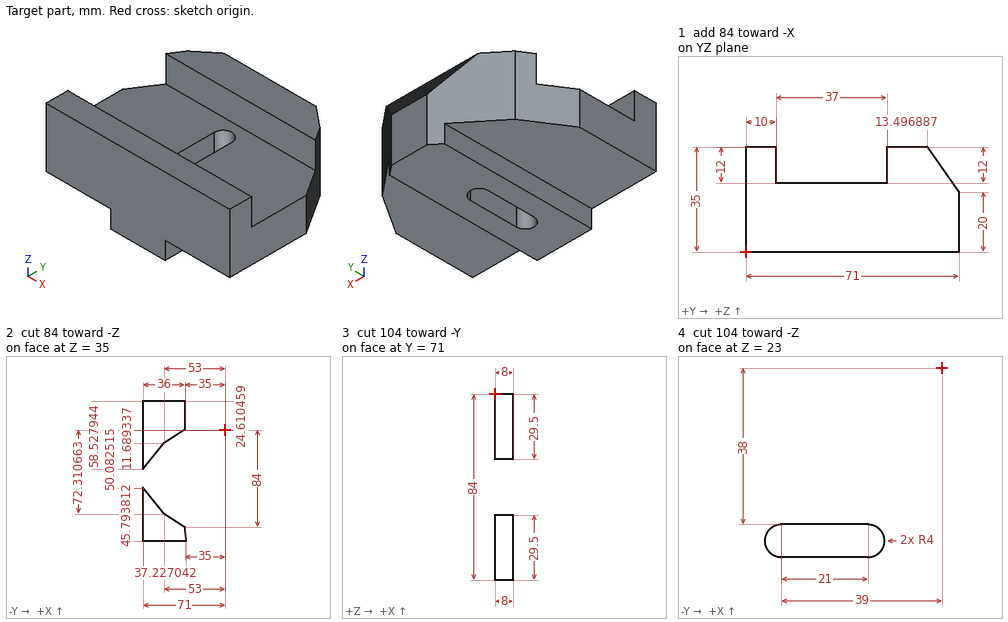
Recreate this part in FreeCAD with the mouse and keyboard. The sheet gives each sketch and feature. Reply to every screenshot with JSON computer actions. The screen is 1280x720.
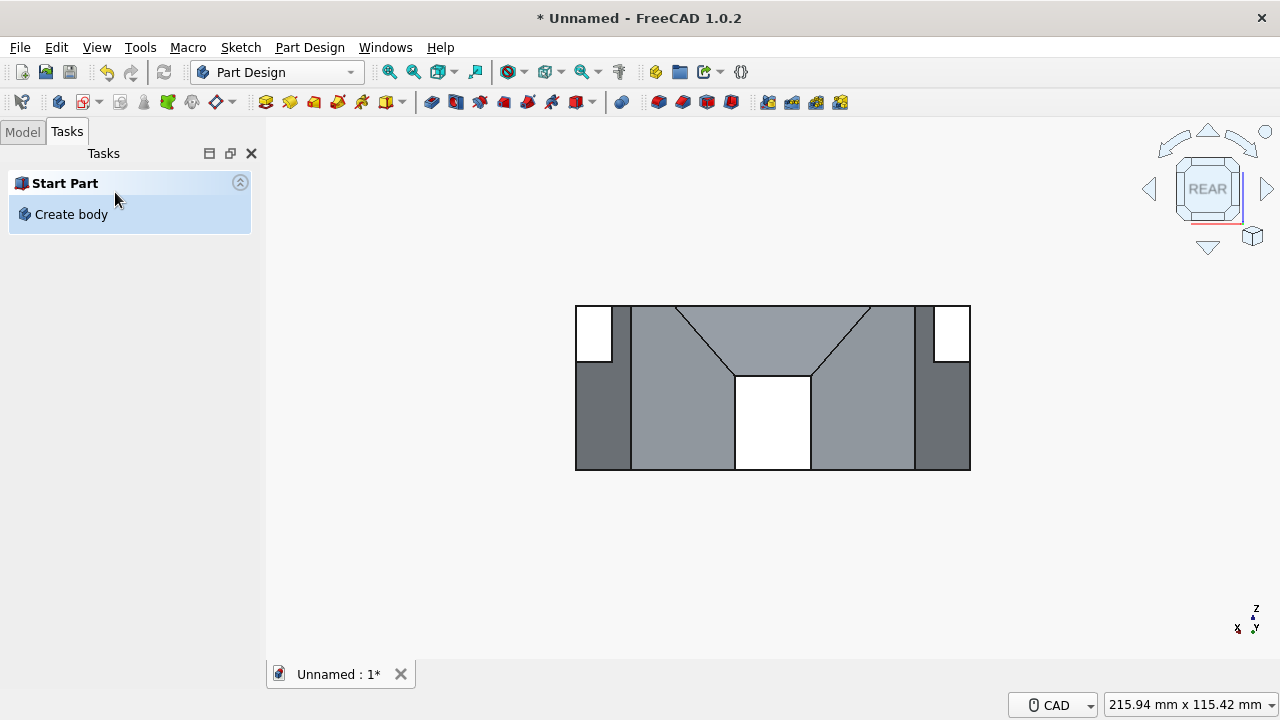
{"action": "left_click", "coordinate": [390, 72]}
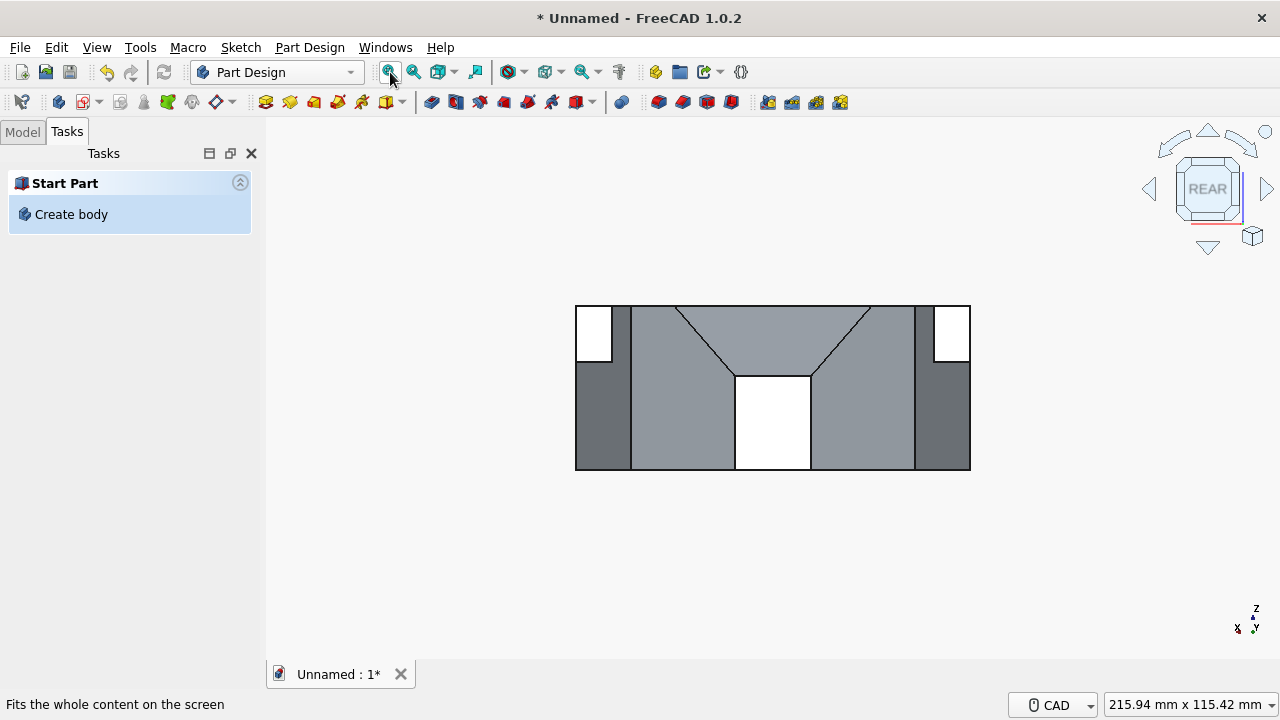
{"action": "left_click", "coordinate": [773, 422]}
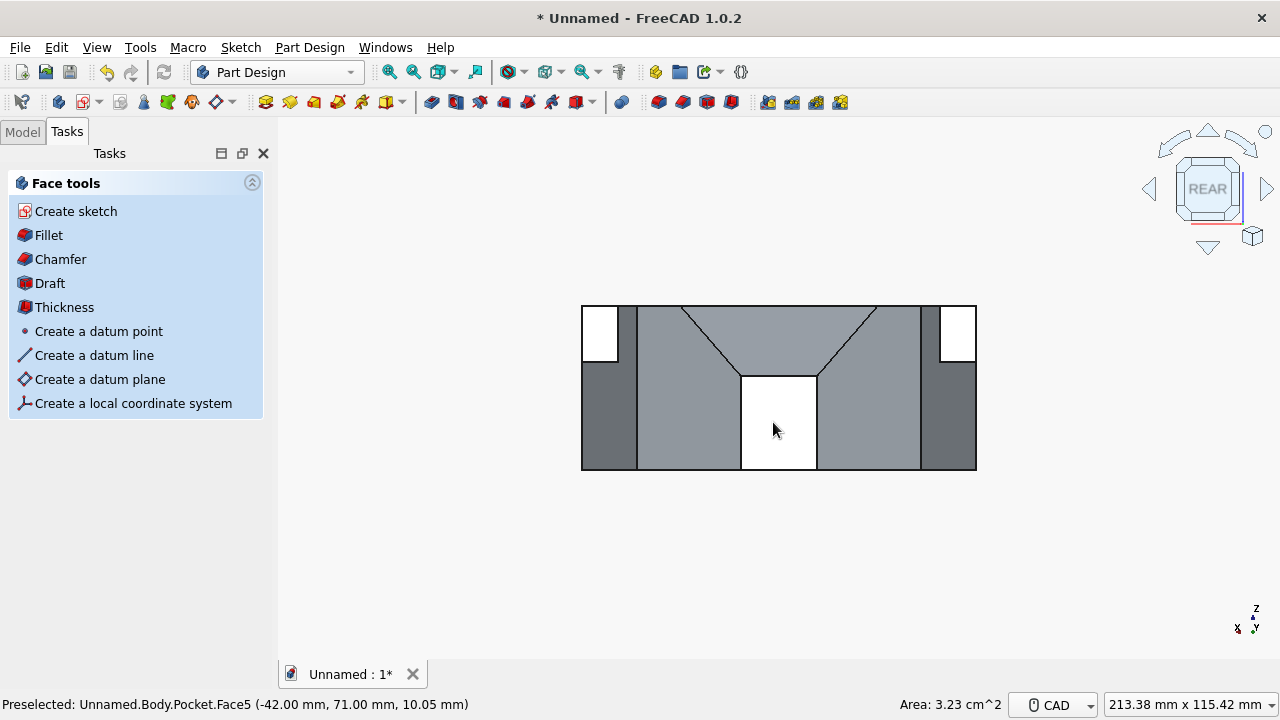
{"action": "left_click", "coordinate": [84, 102]}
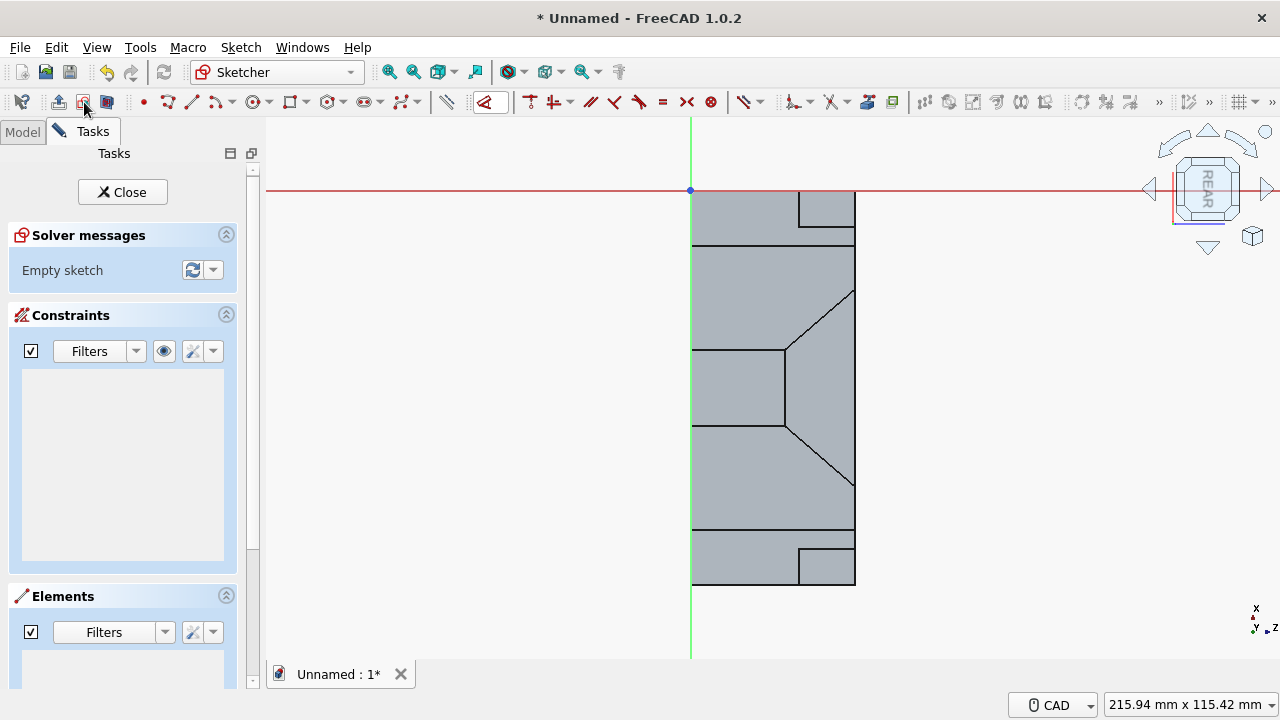
{"action": "left_click", "coordinate": [290, 102]}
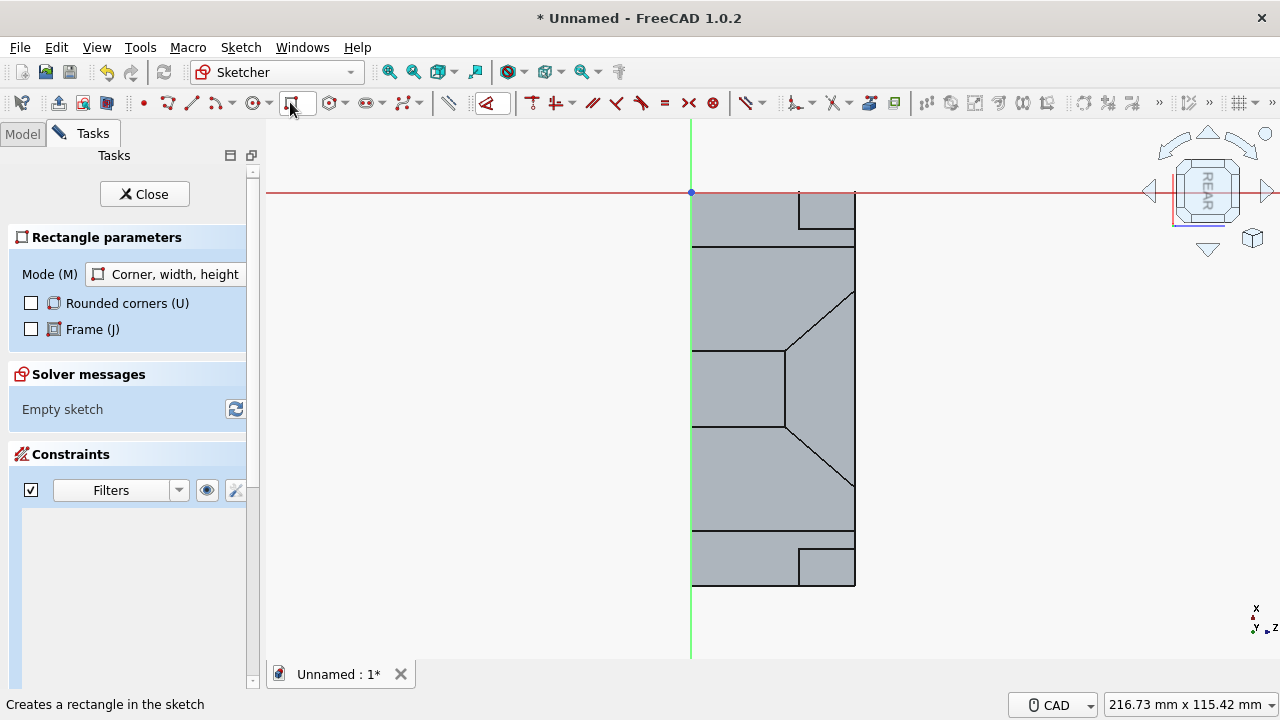
{"action": "left_click", "coordinate": [691, 447]}
{"action": "mouse_move", "coordinate": [729, 585]}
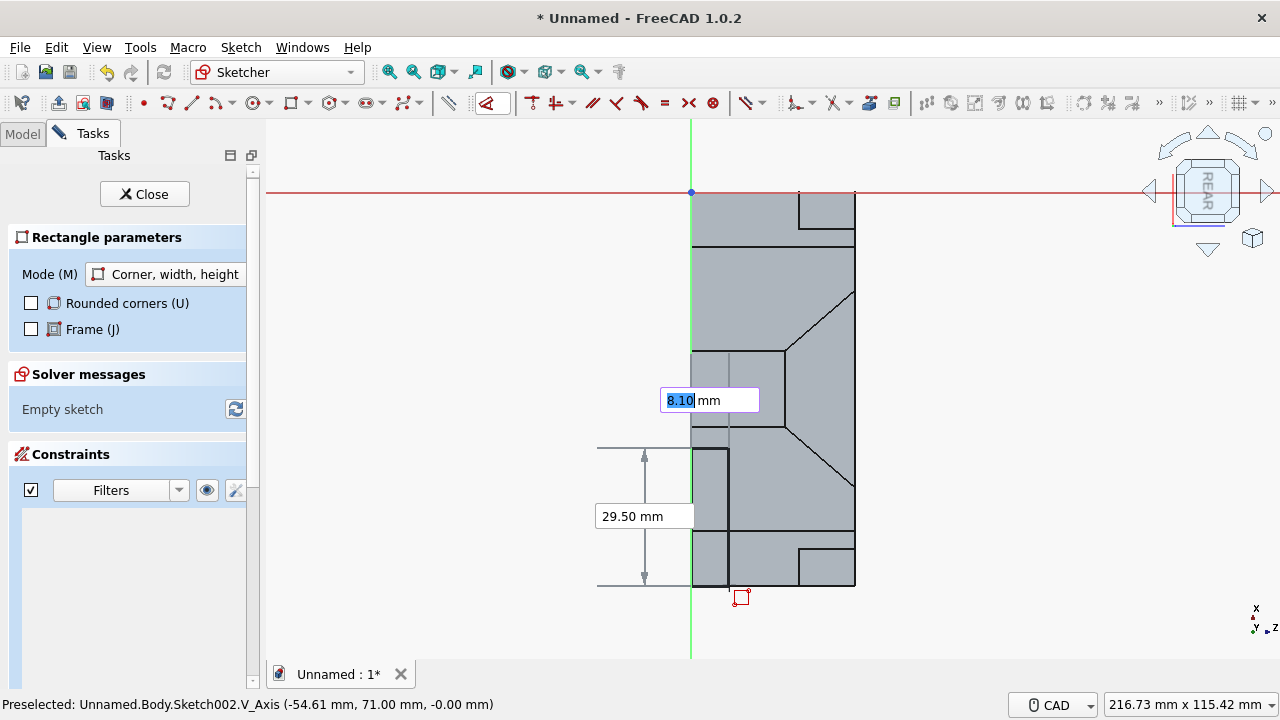
{"action": "type", "text": "8"}
{"action": "key", "text": "Tab"}
{"action": "type", "text": "29.5"}
{"action": "key", "text": "Return"}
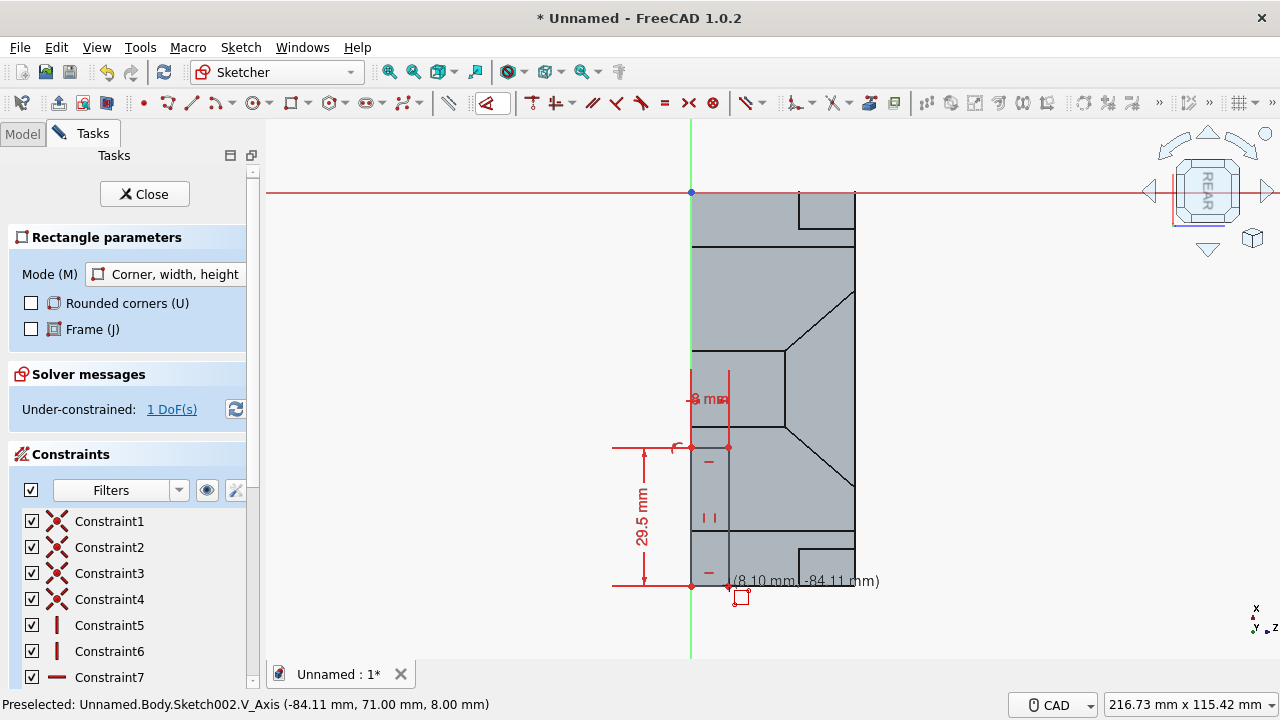
{"action": "left_click", "coordinate": [691, 193]}
{"action": "mouse_move", "coordinate": [729, 331]}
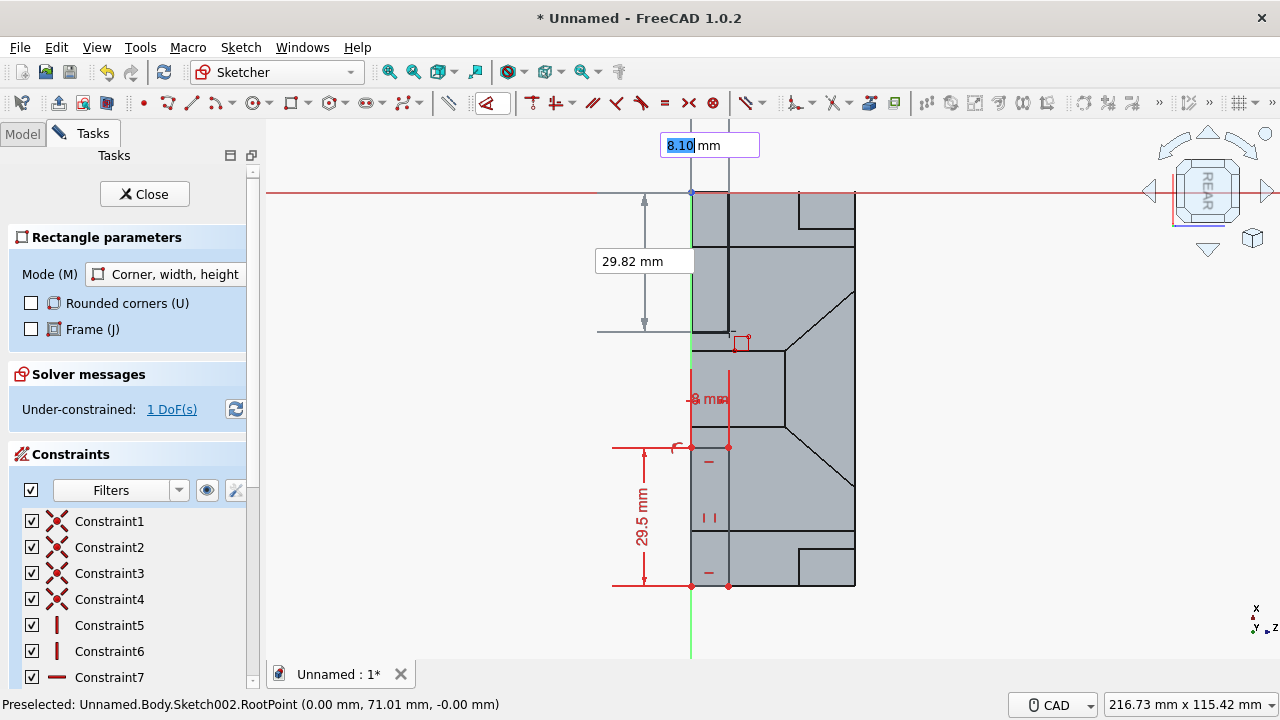
{"action": "type", "text": "8"}
{"action": "key", "text": "Tab"}
{"action": "type", "text": "29.5"}
{"action": "key", "text": "Return"}
{"action": "key", "text": "Escape"}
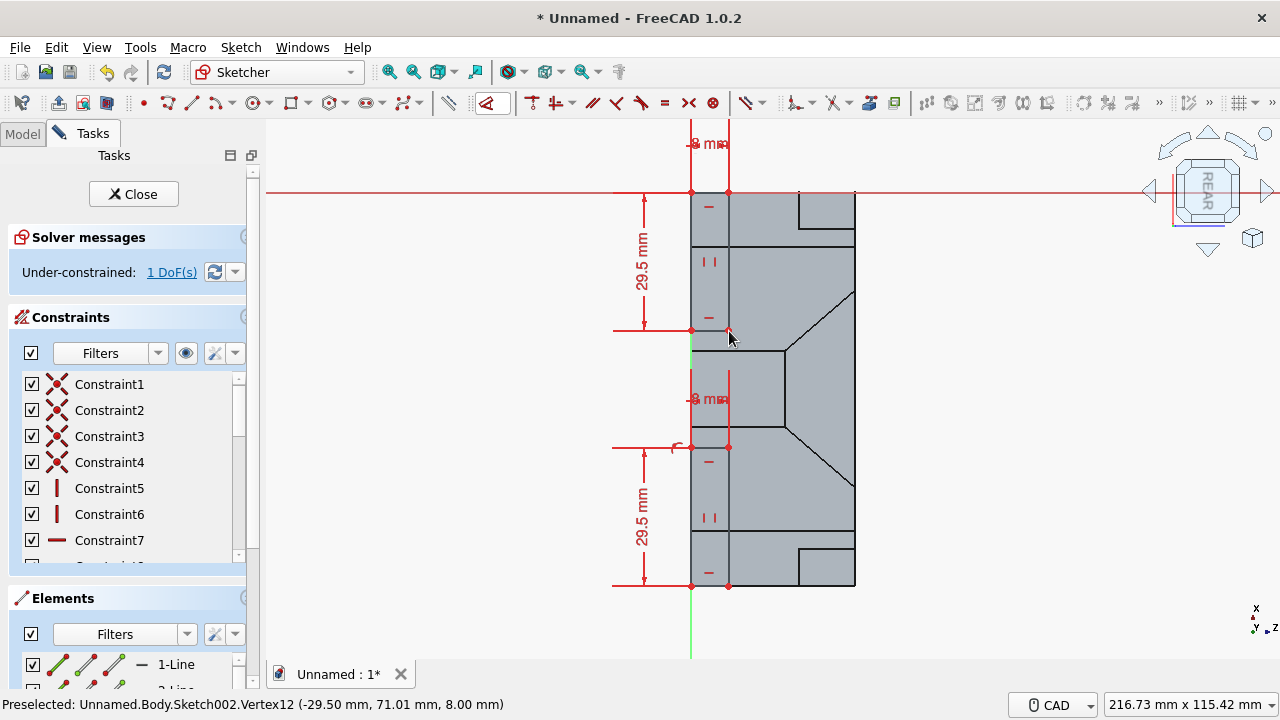
{"action": "left_click", "coordinate": [691, 586]}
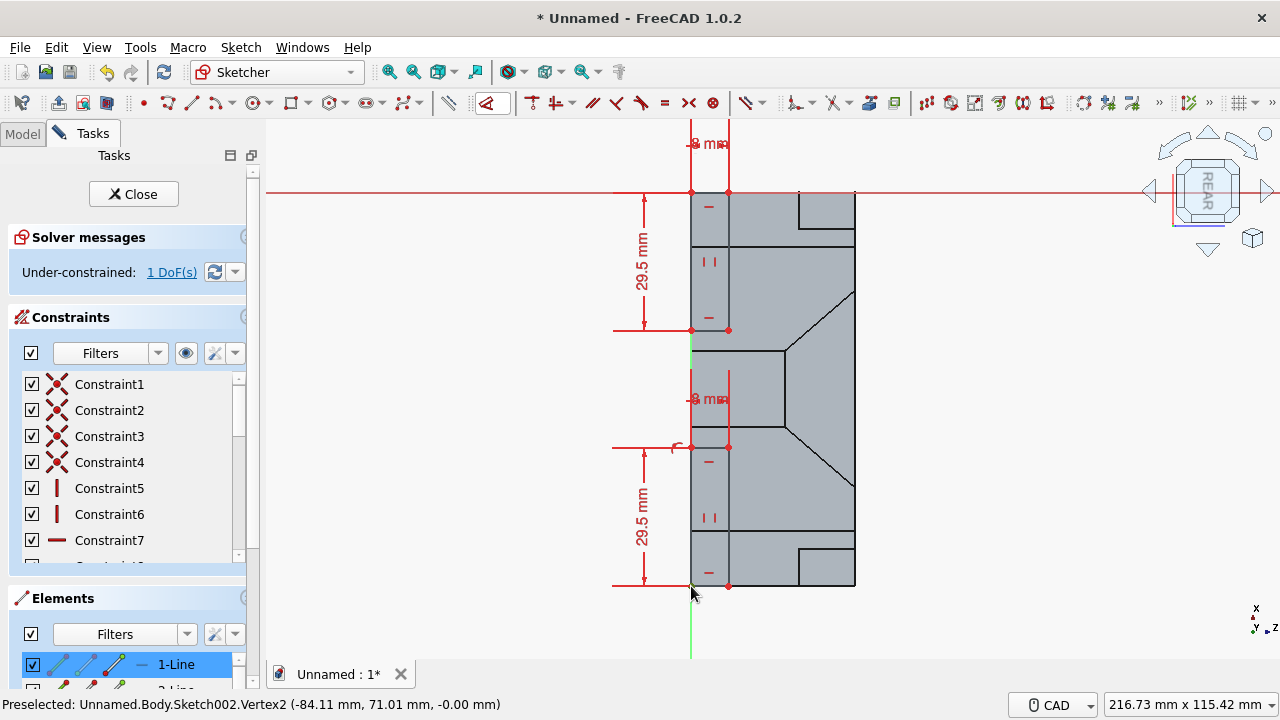
{"action": "key", "text": "i"}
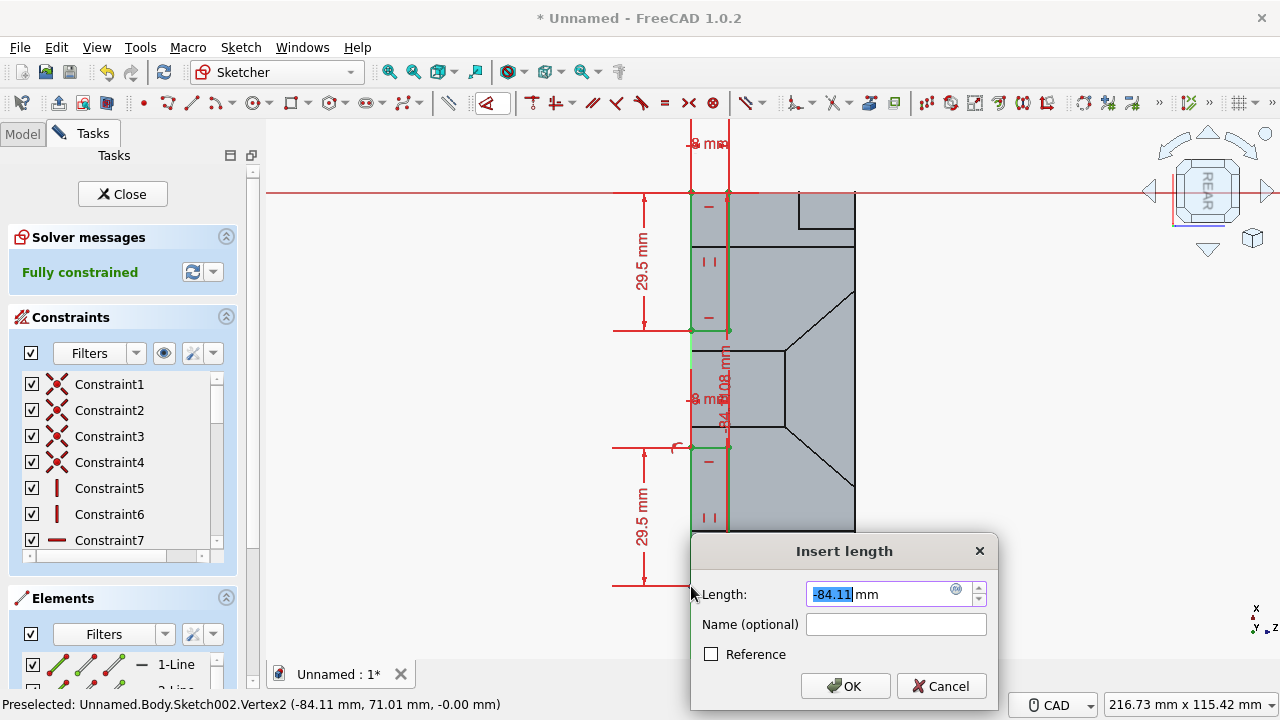
{"action": "type", "text": "-84"}
{"action": "key", "text": "Return"}